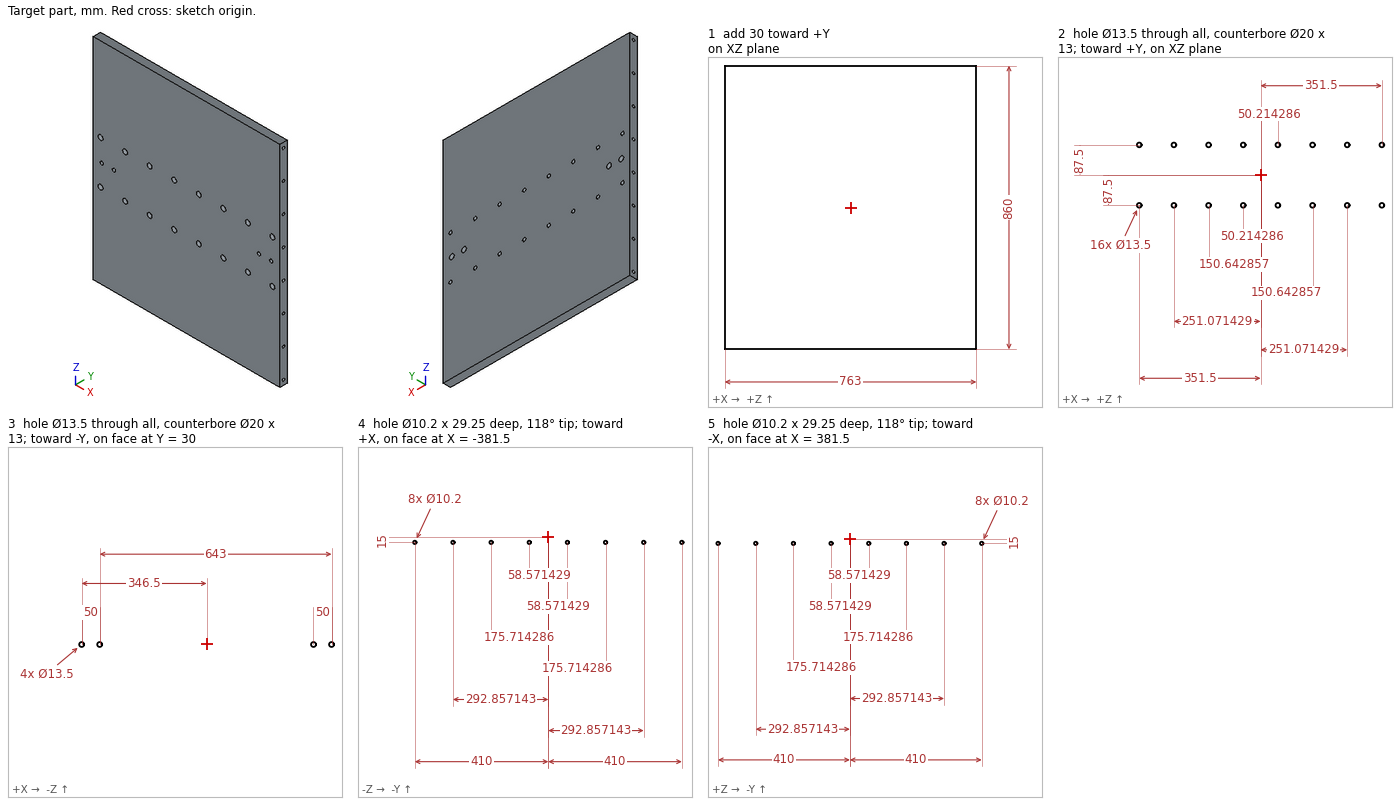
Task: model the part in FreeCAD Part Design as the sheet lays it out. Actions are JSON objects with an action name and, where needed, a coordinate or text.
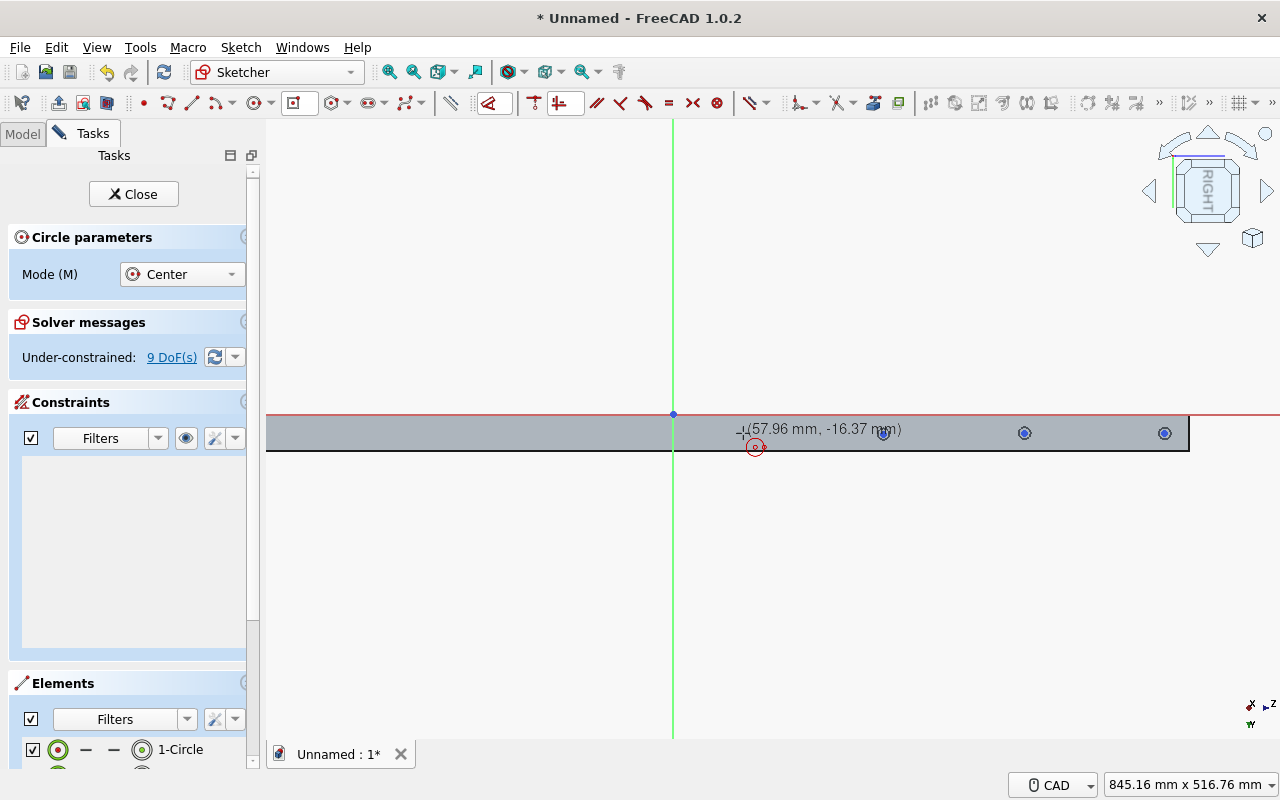
{"action": "left_click", "coordinate": [743, 433]}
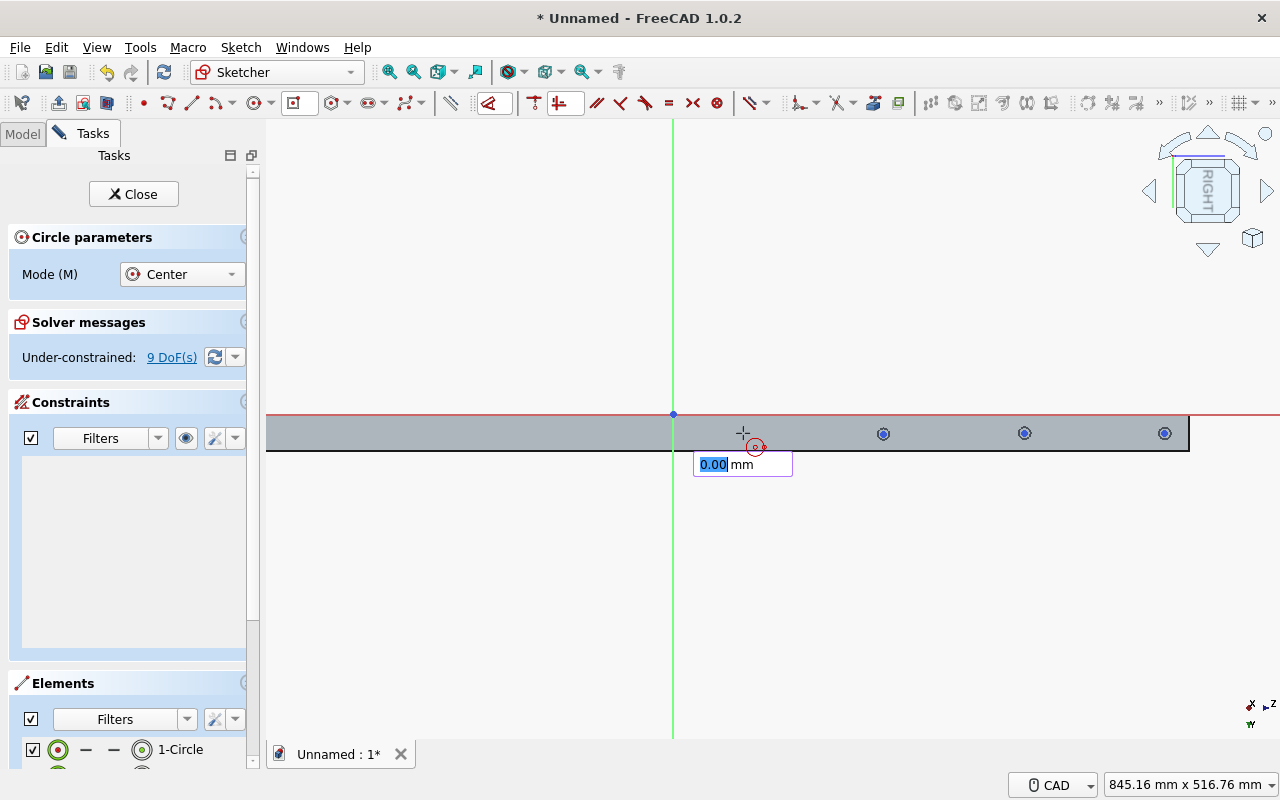
{"action": "scroll", "coordinate": [748, 437], "scroll_direction": "up", "scroll_amount": 5}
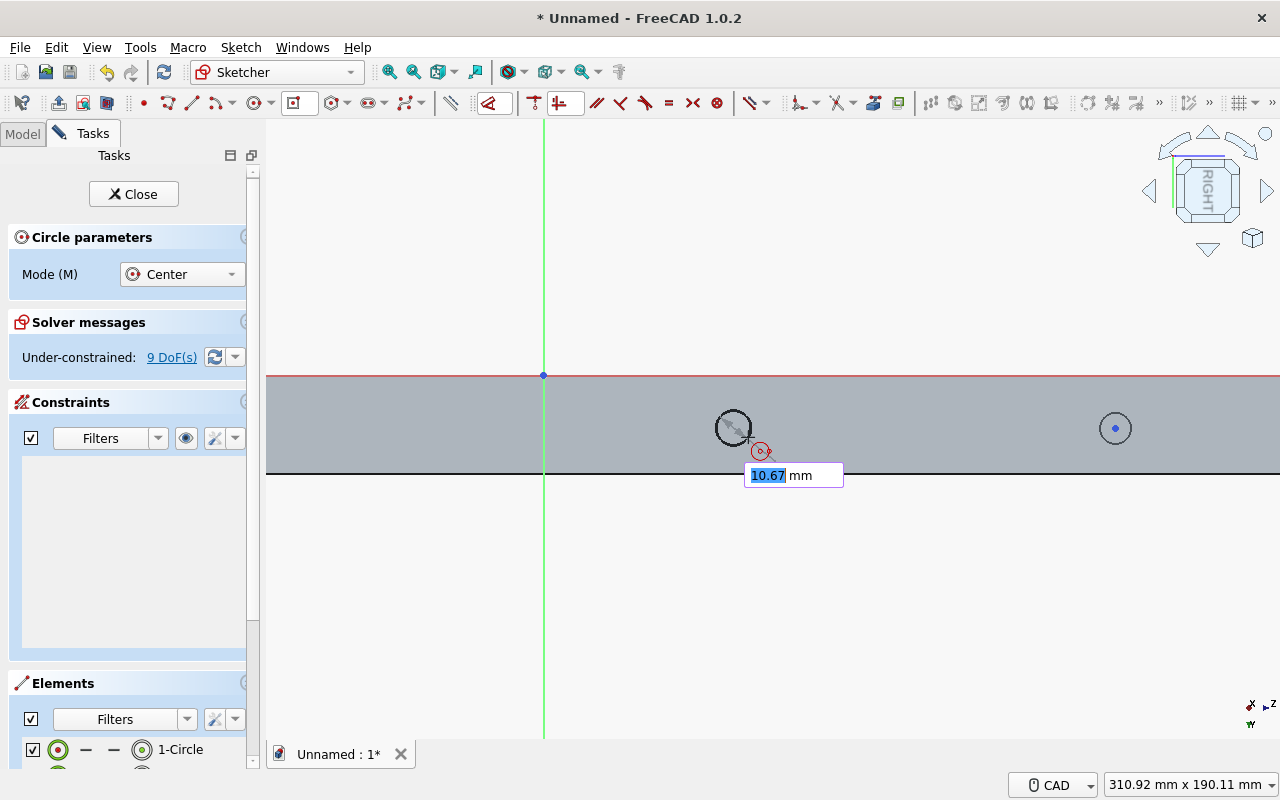
{"action": "left_click", "coordinate": [746, 436]}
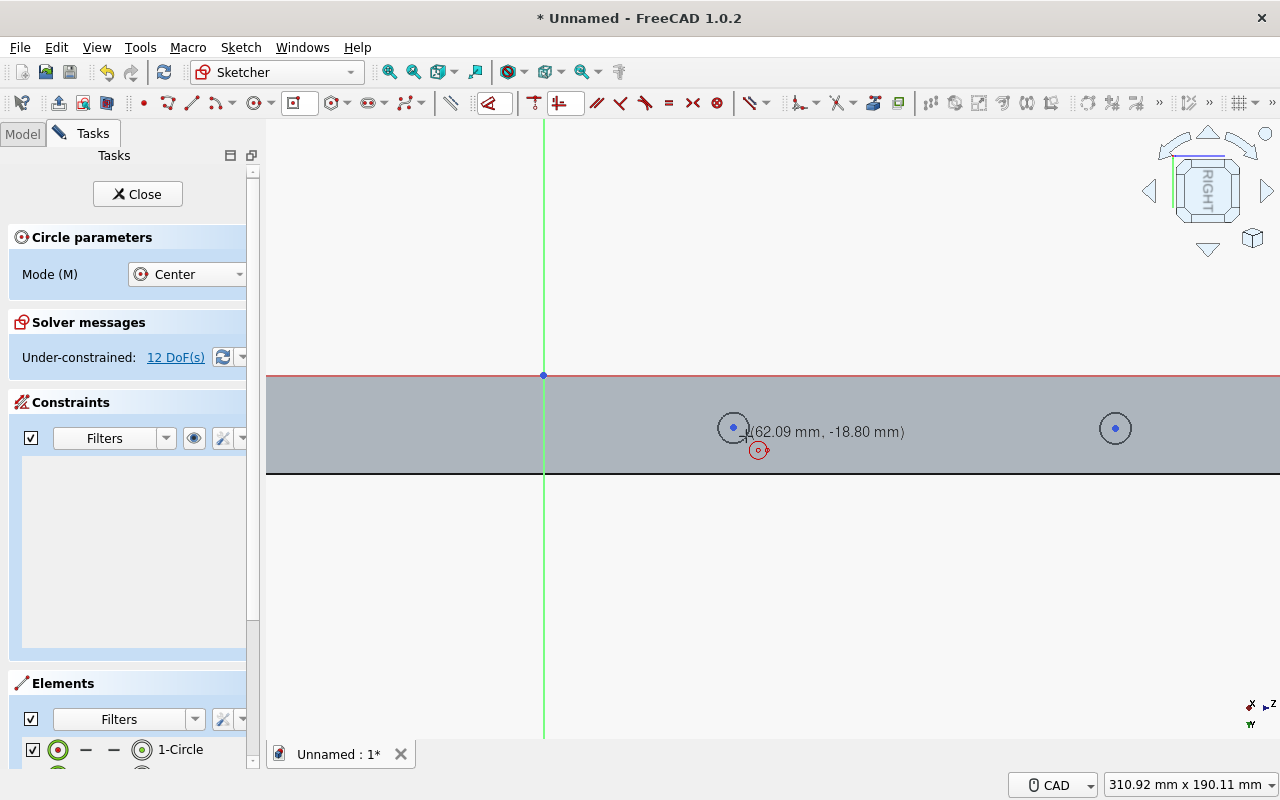
{"action": "scroll", "coordinate": [352, 425], "scroll_direction": "up", "scroll_amount": 2}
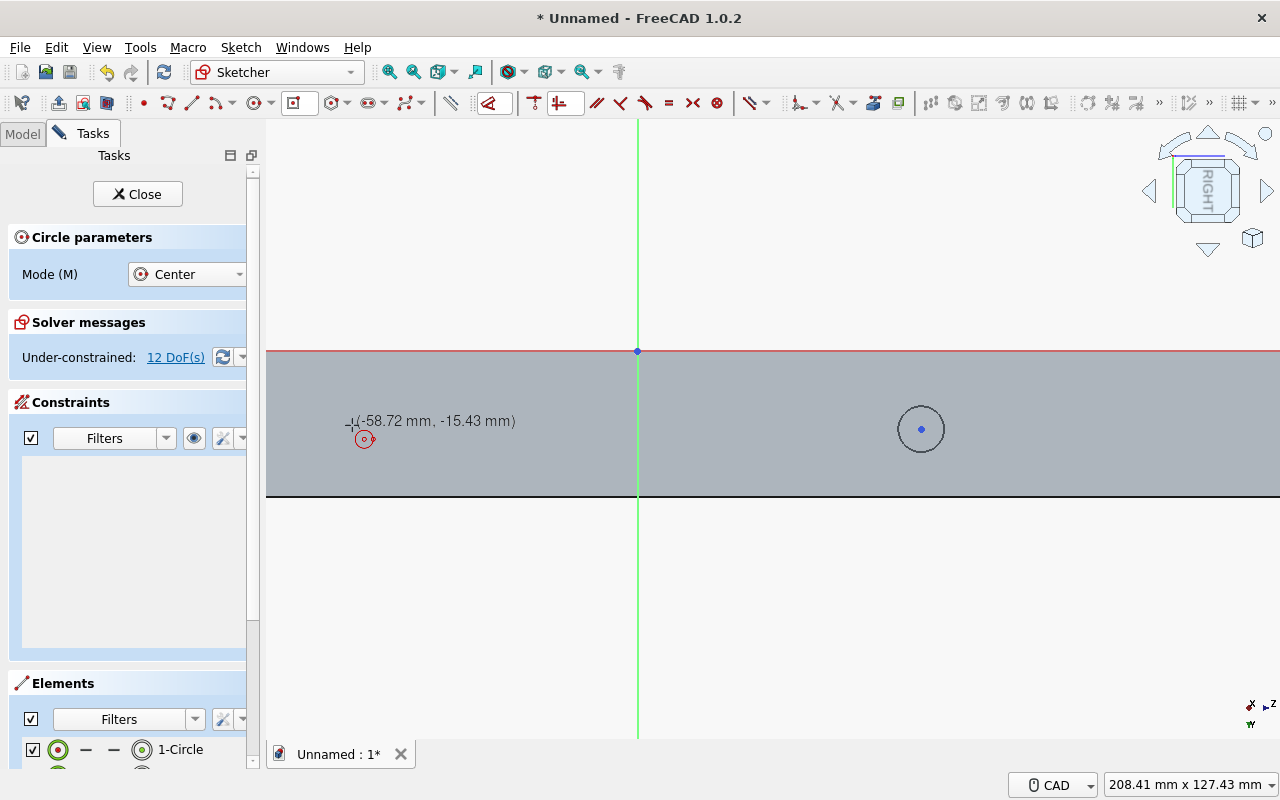
{"action": "scroll", "coordinate": [715, 434], "scroll_direction": "down", "scroll_amount": 10}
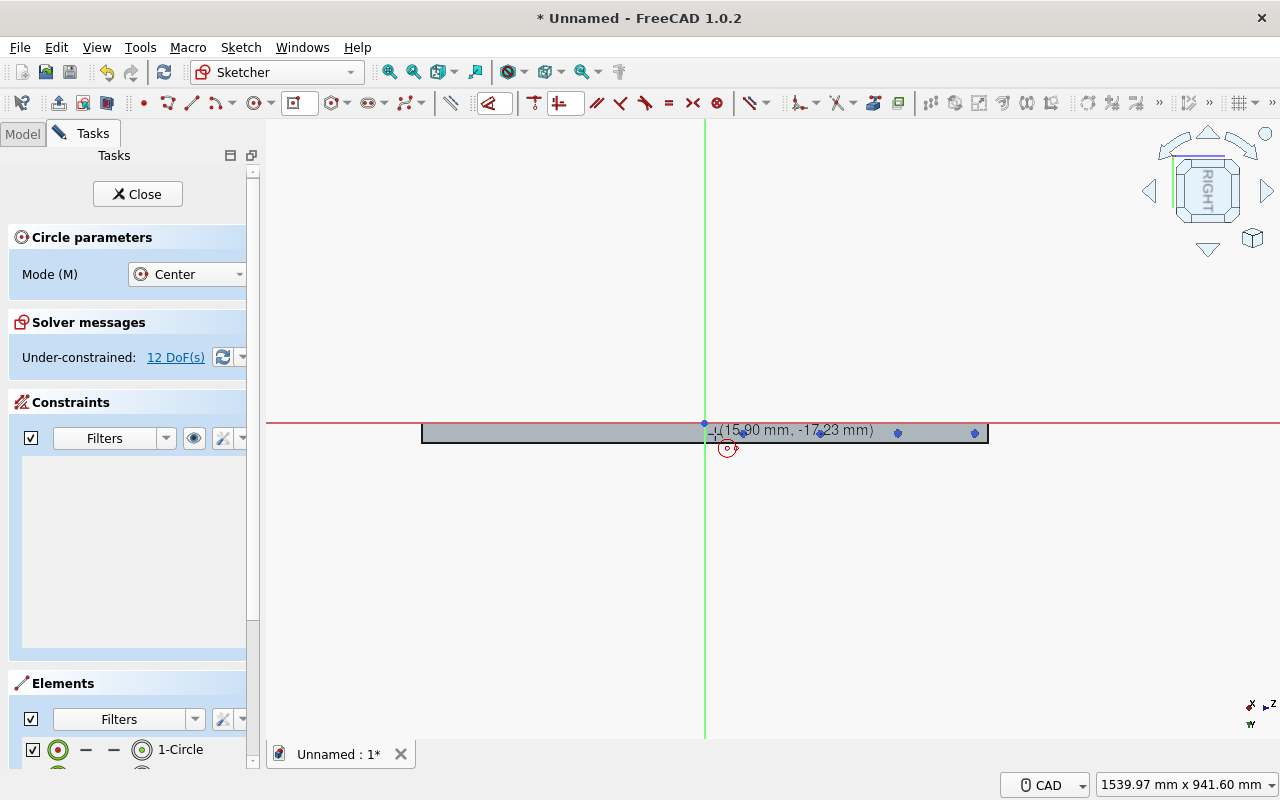
{"action": "scroll", "coordinate": [666, 433], "scroll_direction": "up", "scroll_amount": 3}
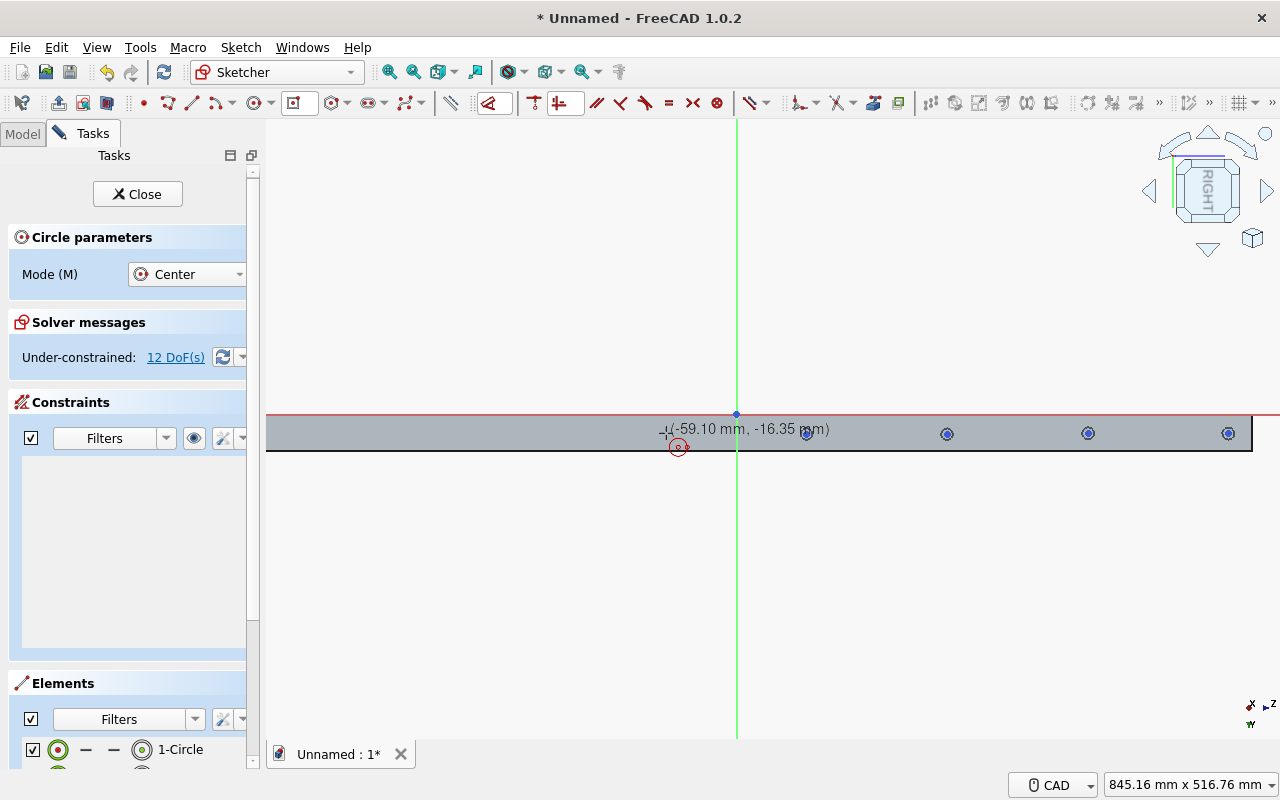
{"action": "left_click", "coordinate": [666, 433]}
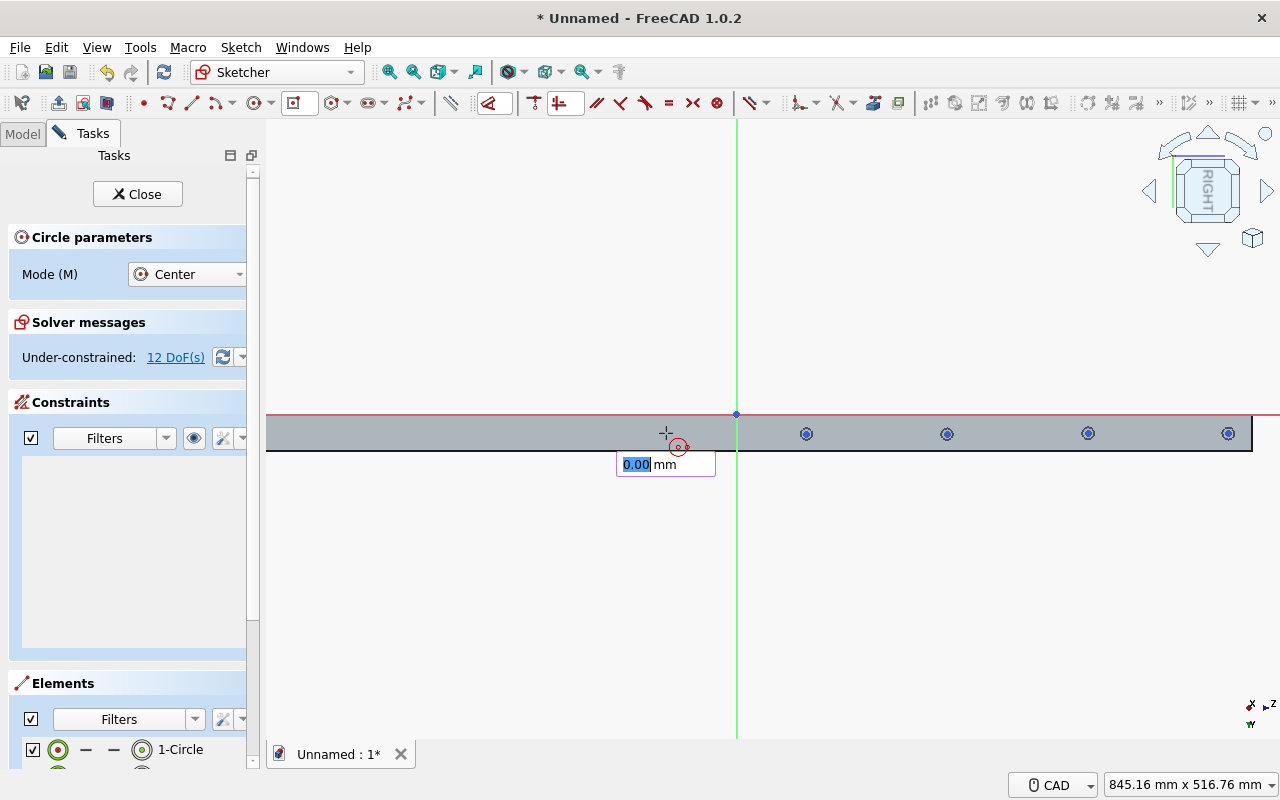
{"action": "scroll", "coordinate": [671, 437], "scroll_direction": "up", "scroll_amount": 5}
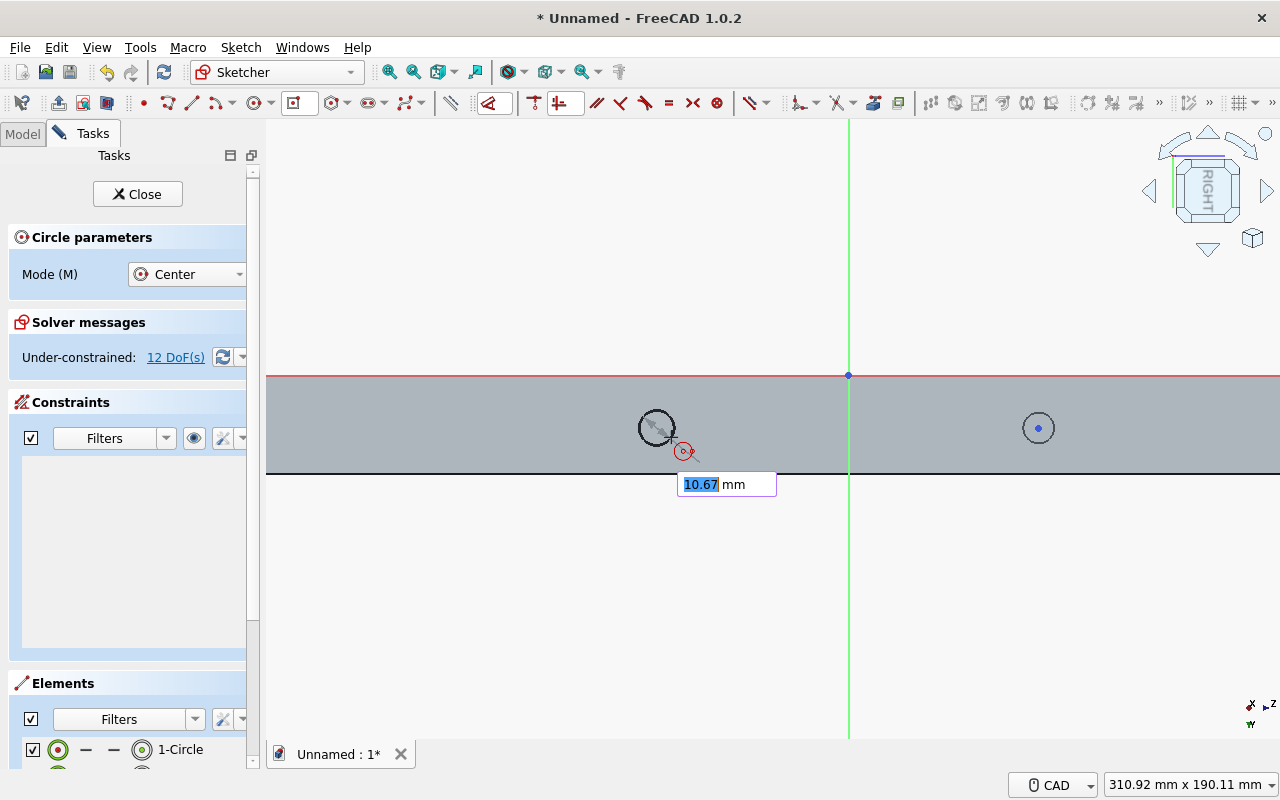
{"action": "left_click", "coordinate": [669, 436]}